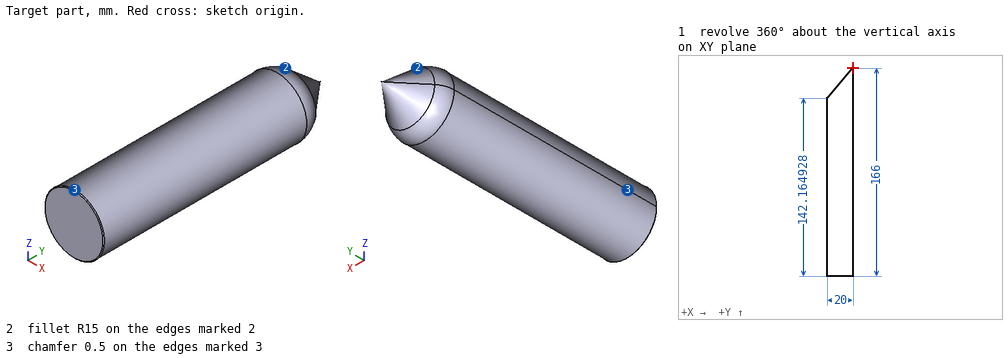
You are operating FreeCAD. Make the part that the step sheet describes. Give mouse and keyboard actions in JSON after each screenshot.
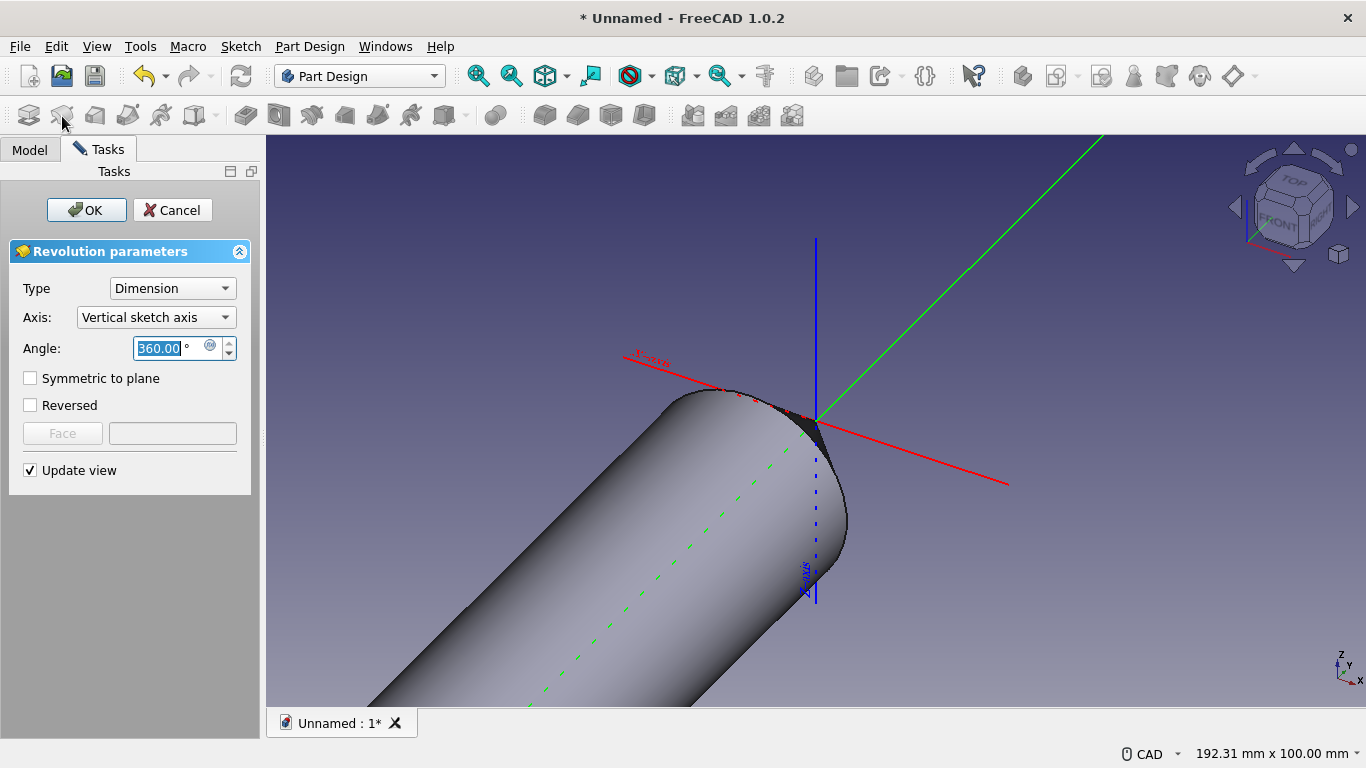
{"action": "left_click", "coordinate": [87, 210]}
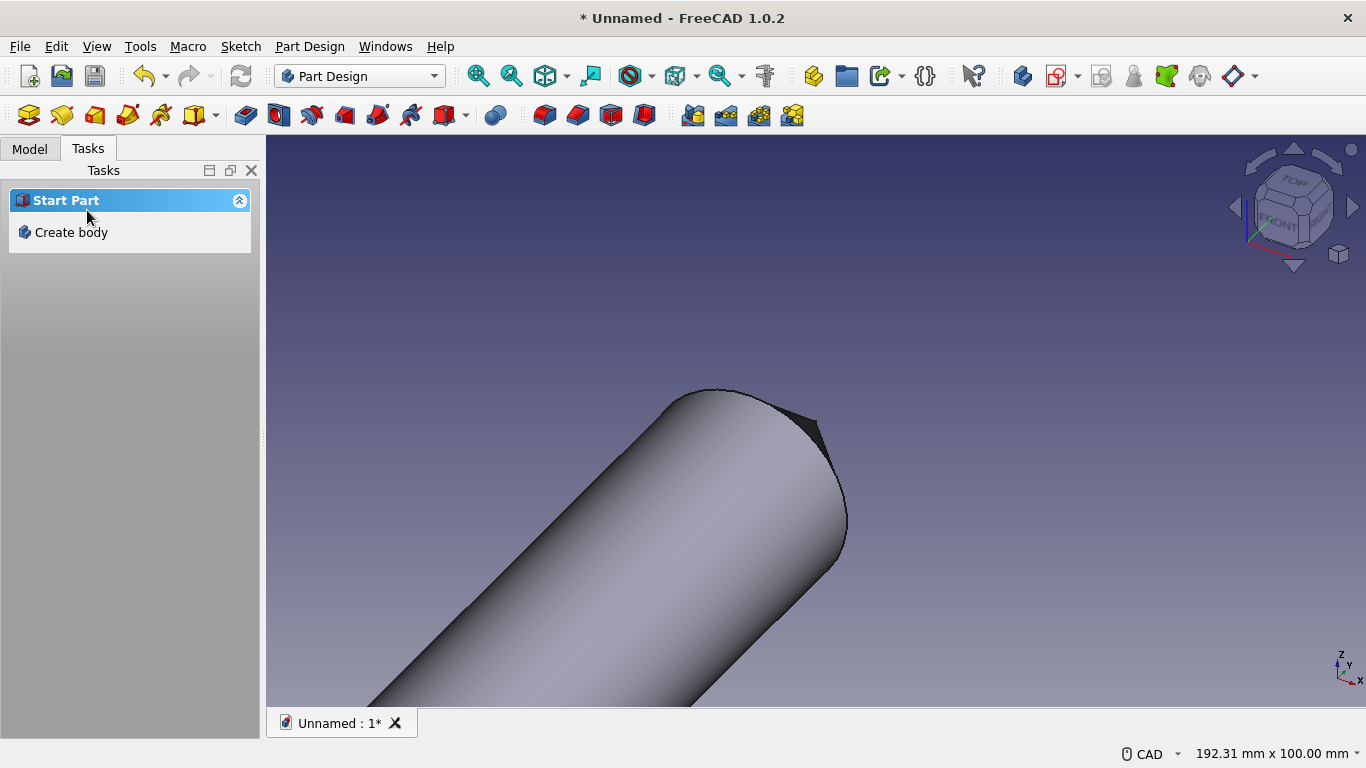
{"action": "left_click", "coordinate": [479, 76]}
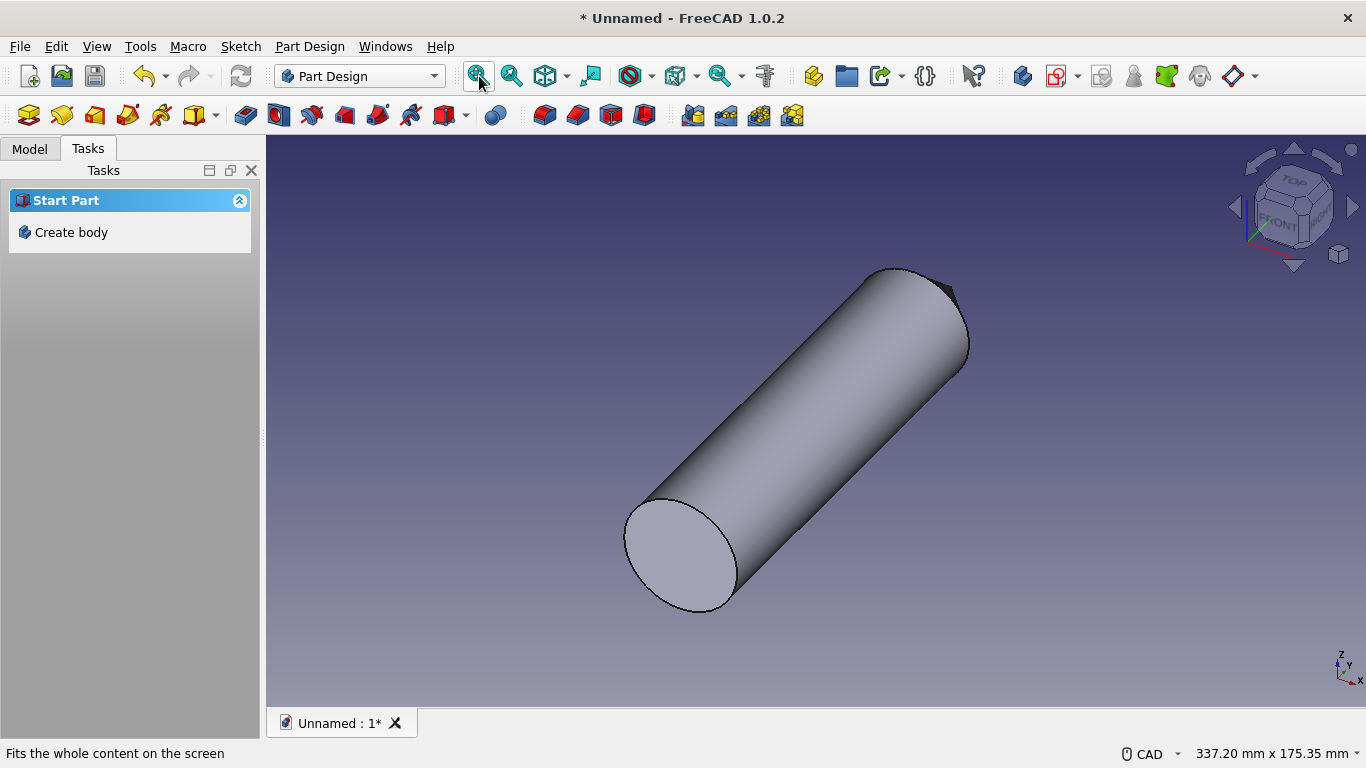
{"action": "key", "text": "0"}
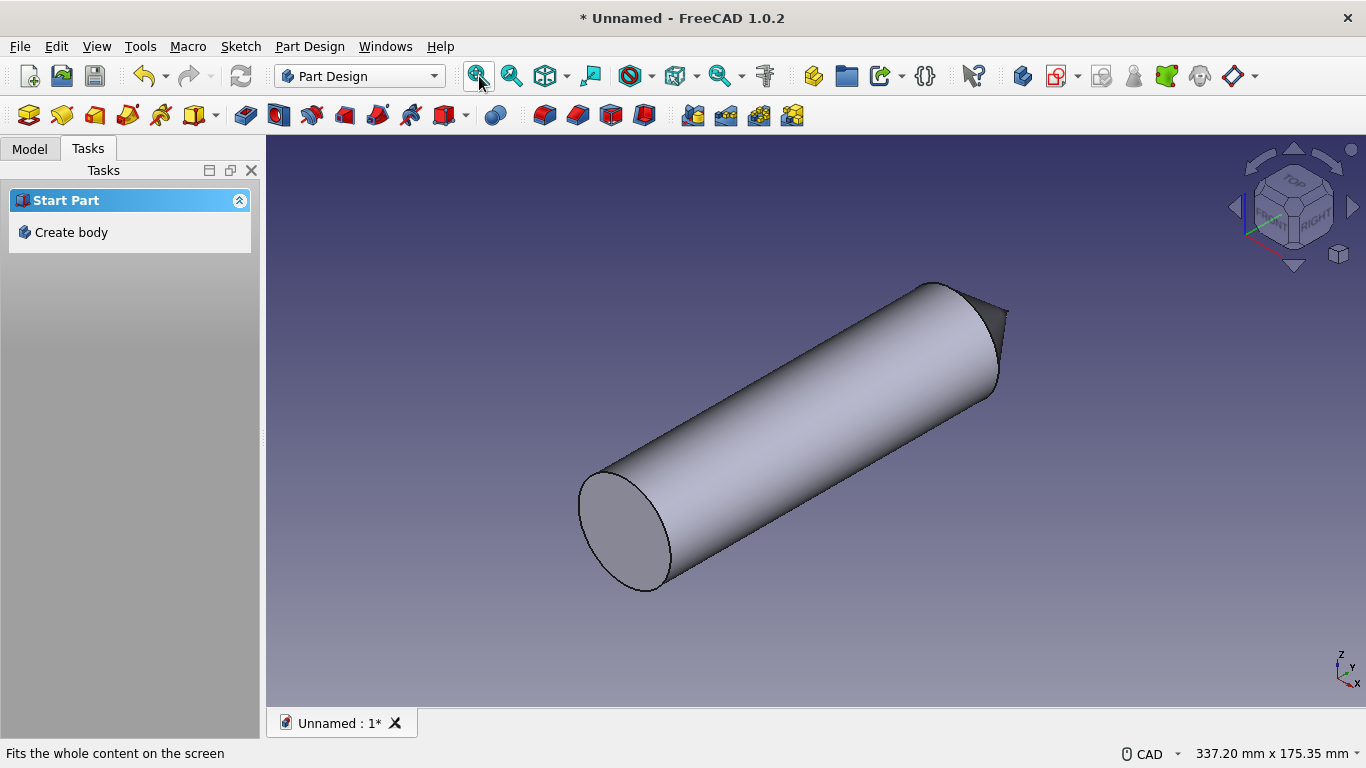
{"action": "key", "text": "2"}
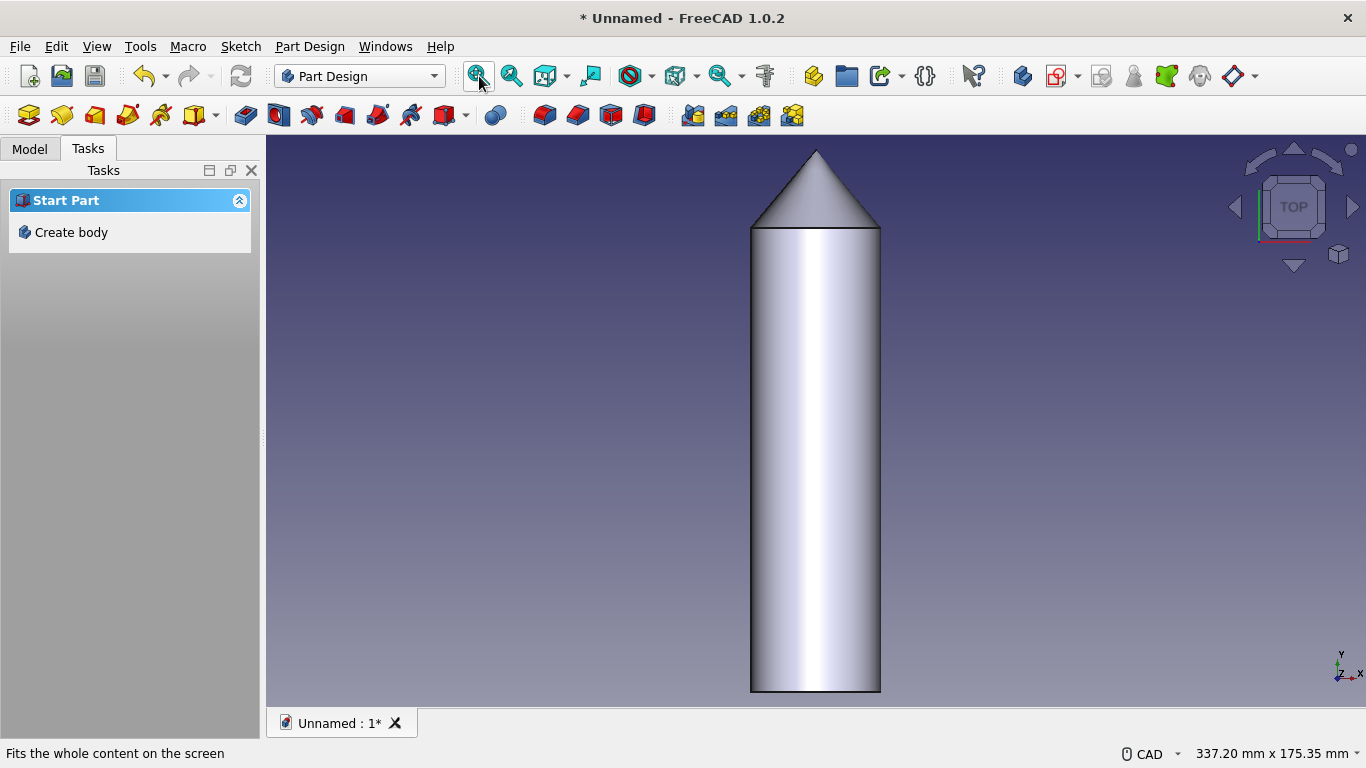
{"action": "left_click", "coordinate": [869, 227]}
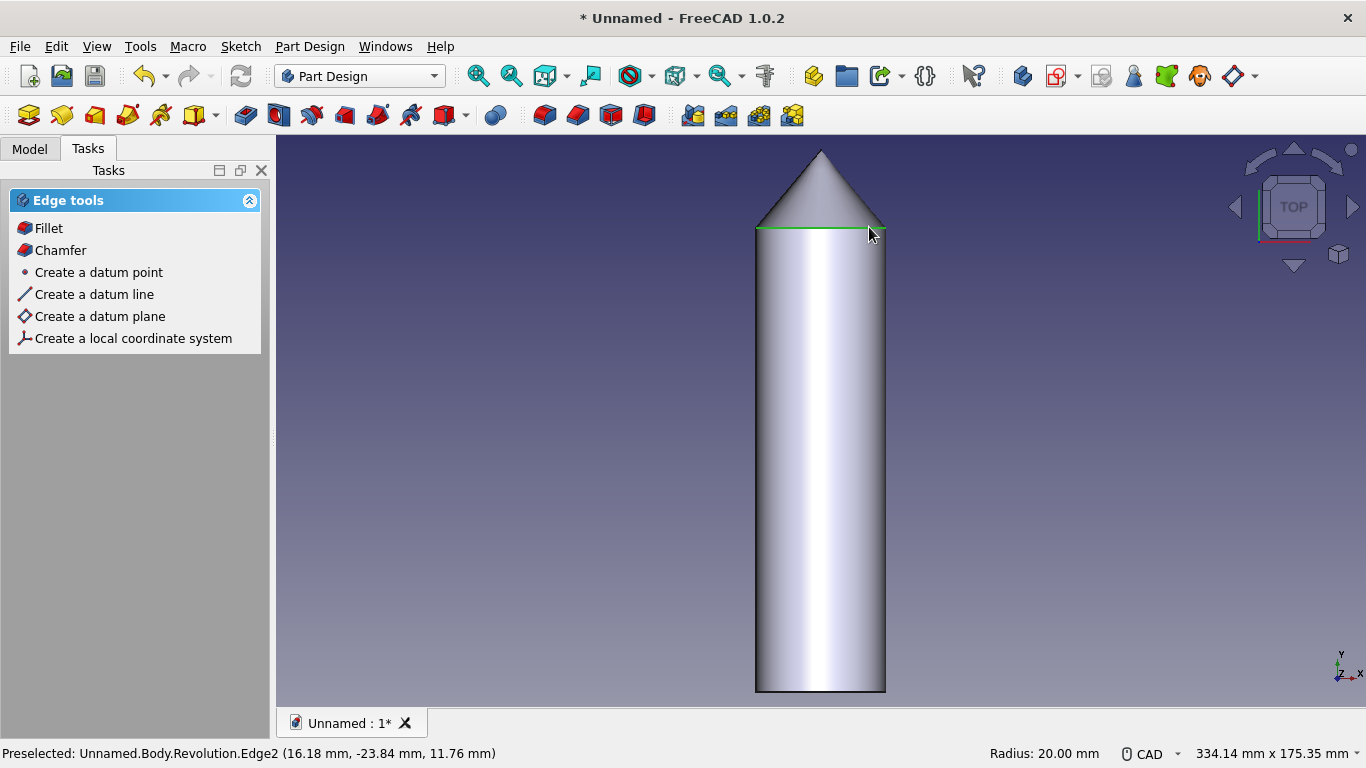
{"action": "left_click", "coordinate": [545, 116]}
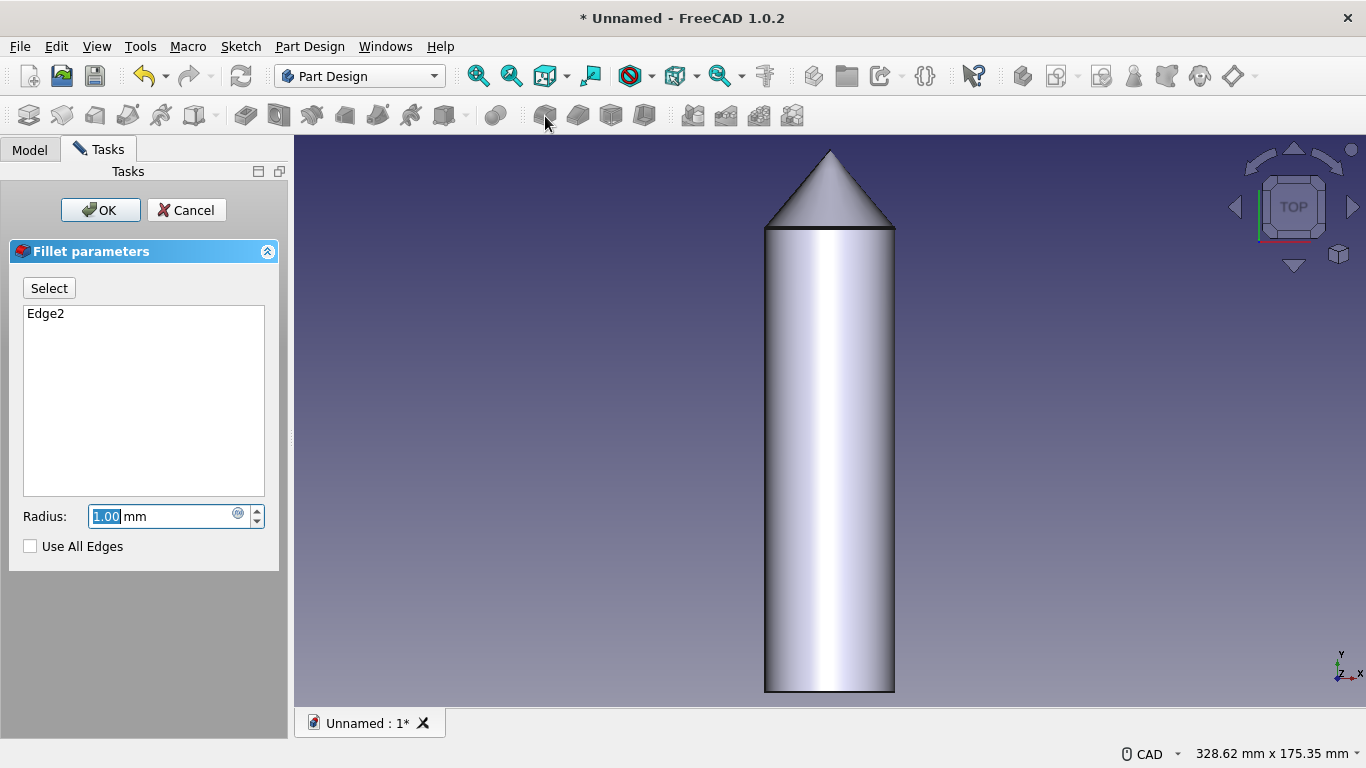
{"action": "type", "text": "15"}
{"action": "key", "text": "Tab"}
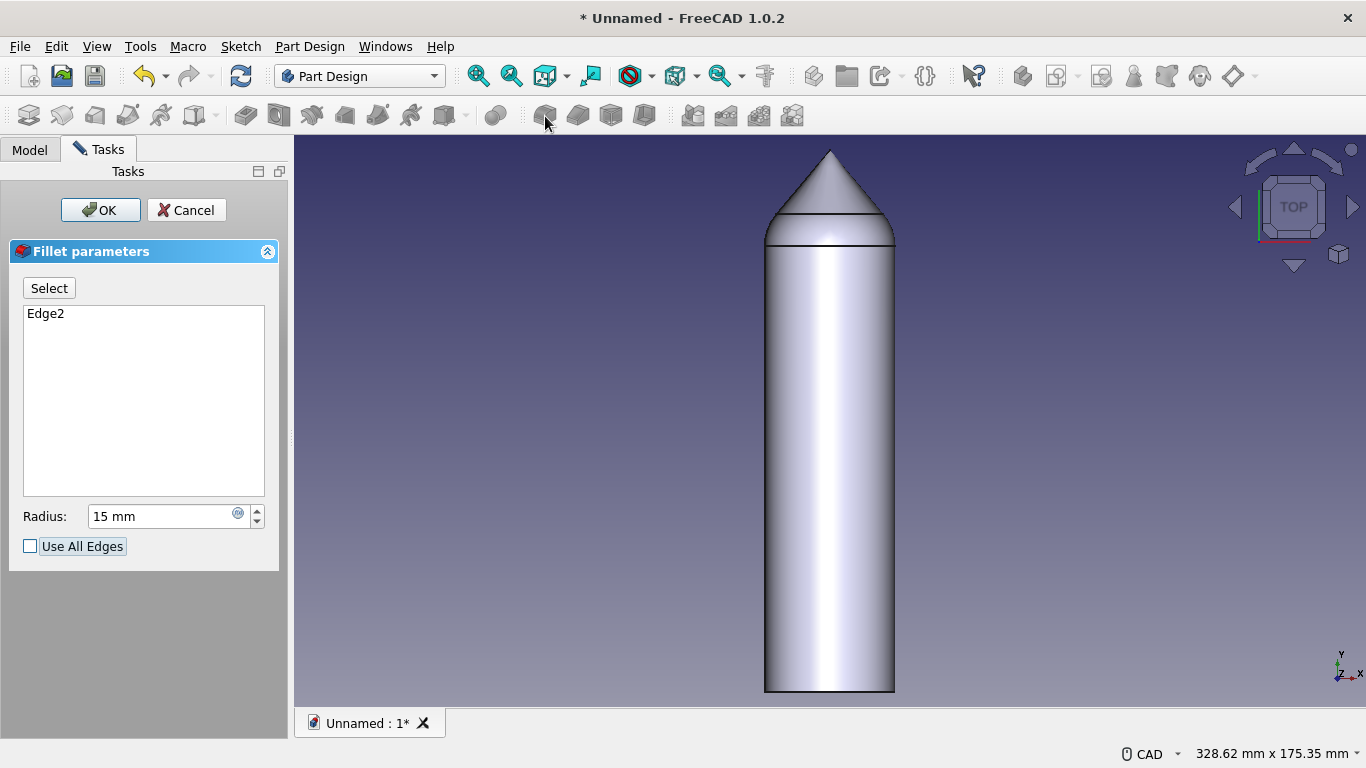
{"action": "left_click", "coordinate": [101, 210]}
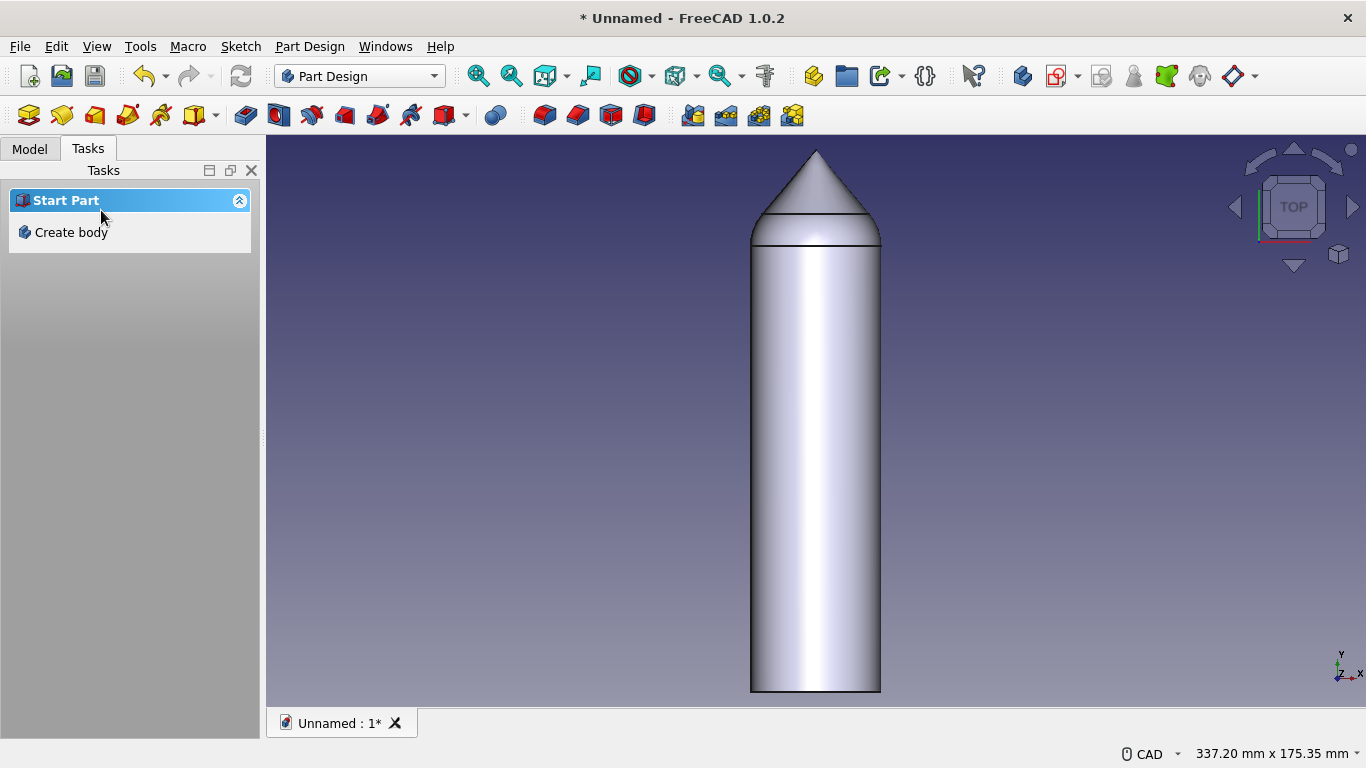
{"action": "key", "text": "0"}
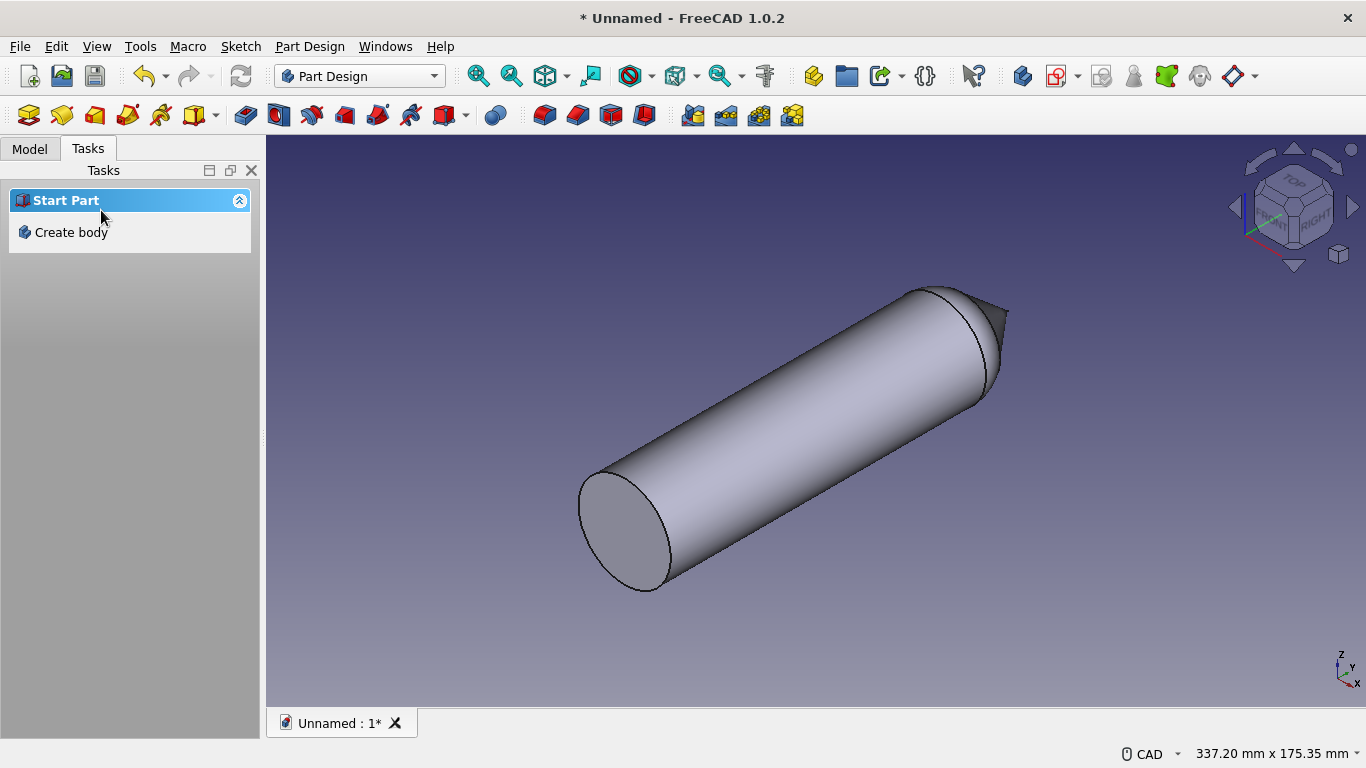
{"action": "left_click", "coordinate": [671, 557]}